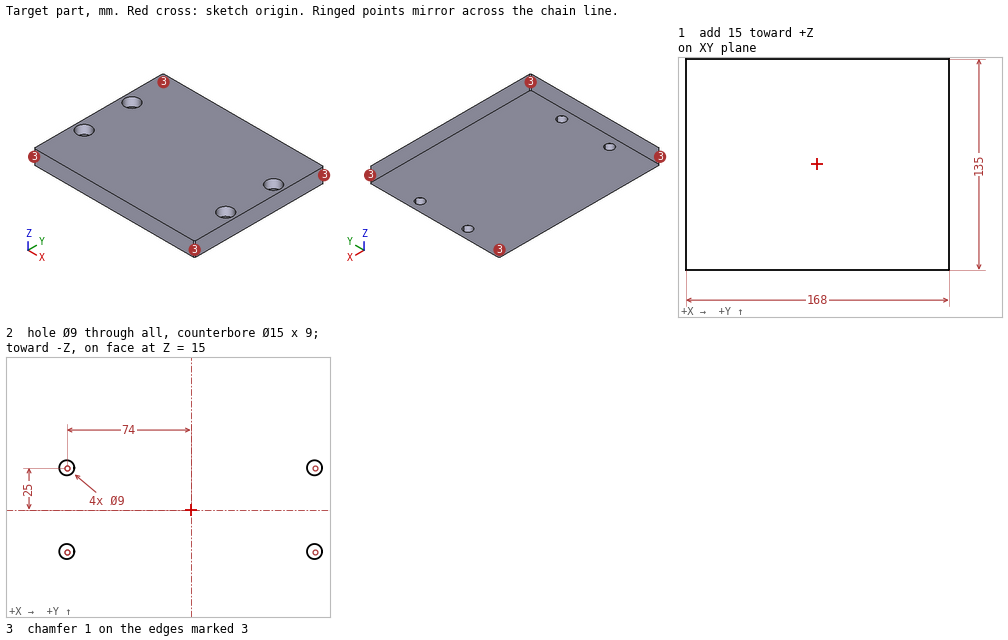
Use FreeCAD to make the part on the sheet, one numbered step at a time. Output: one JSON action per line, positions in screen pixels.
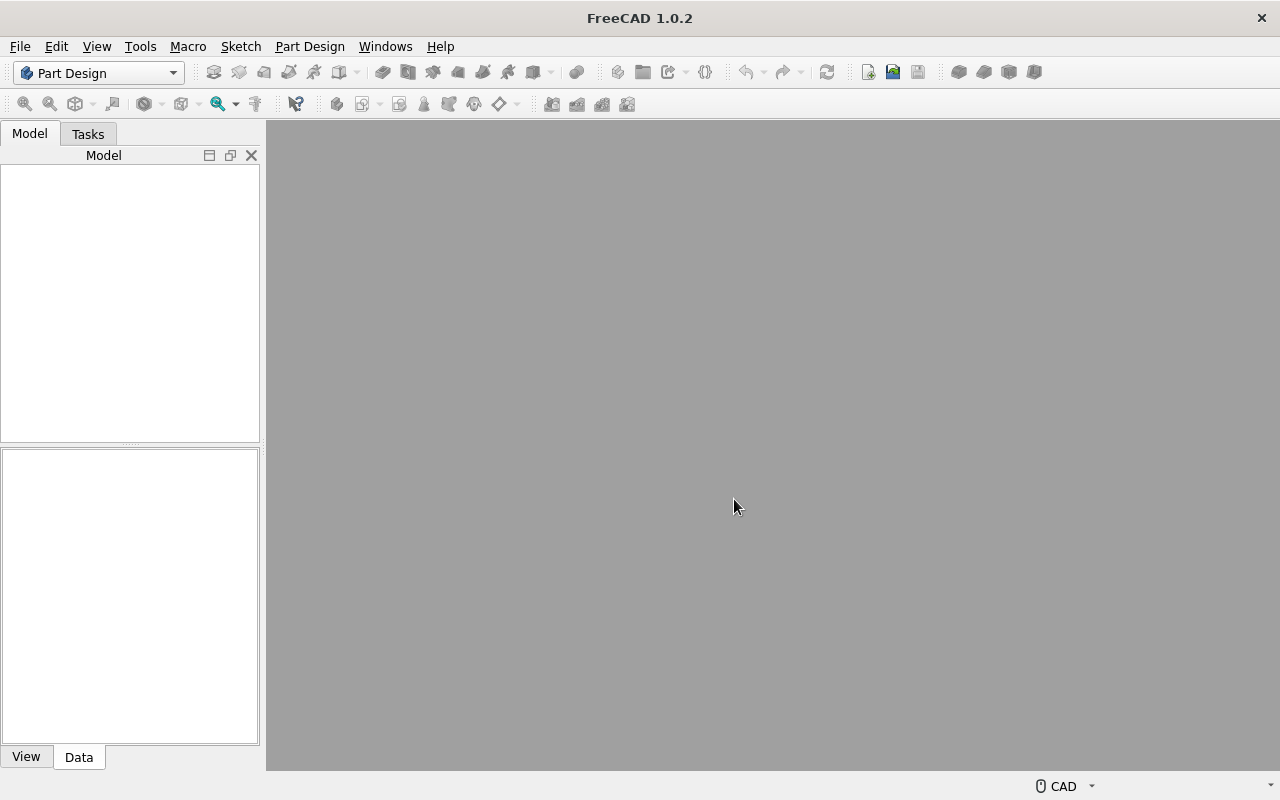
{"action": "key", "text": "ctrl+n"}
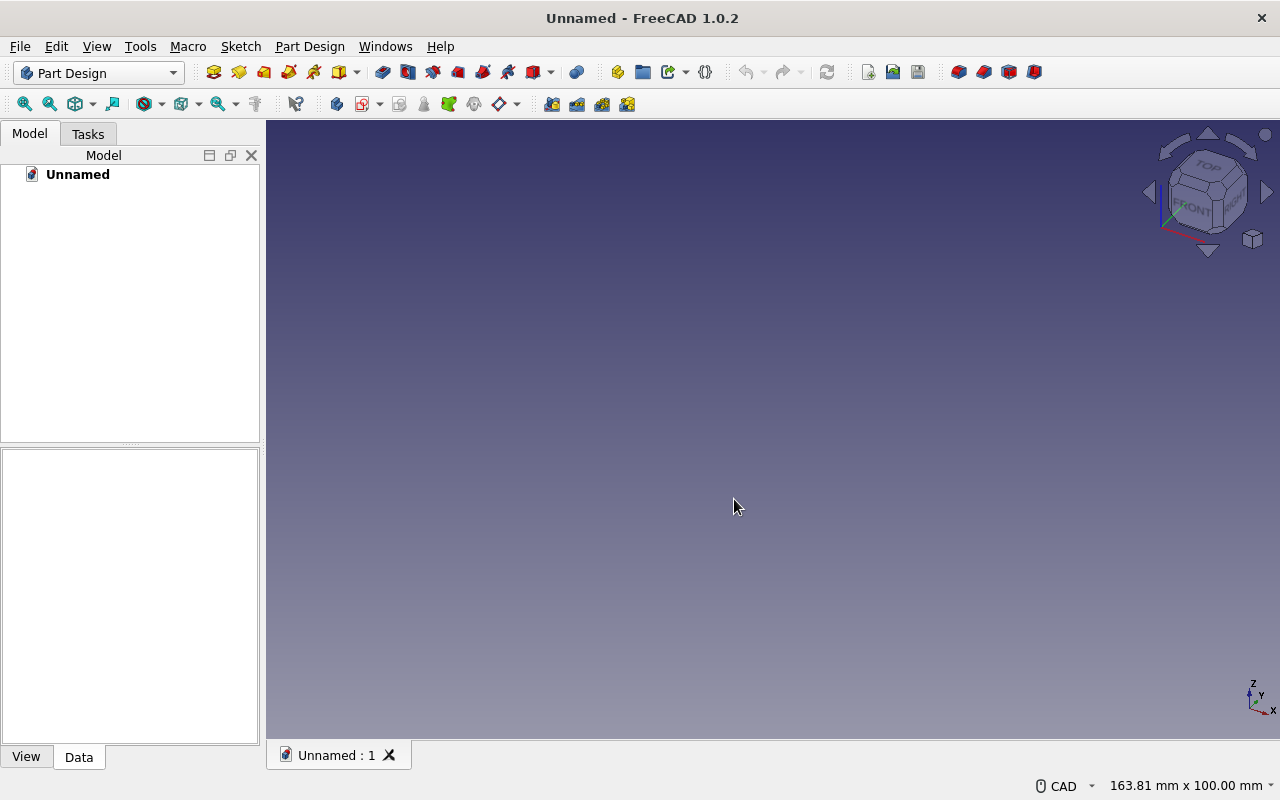
{"action": "left_click", "coordinate": [362, 104]}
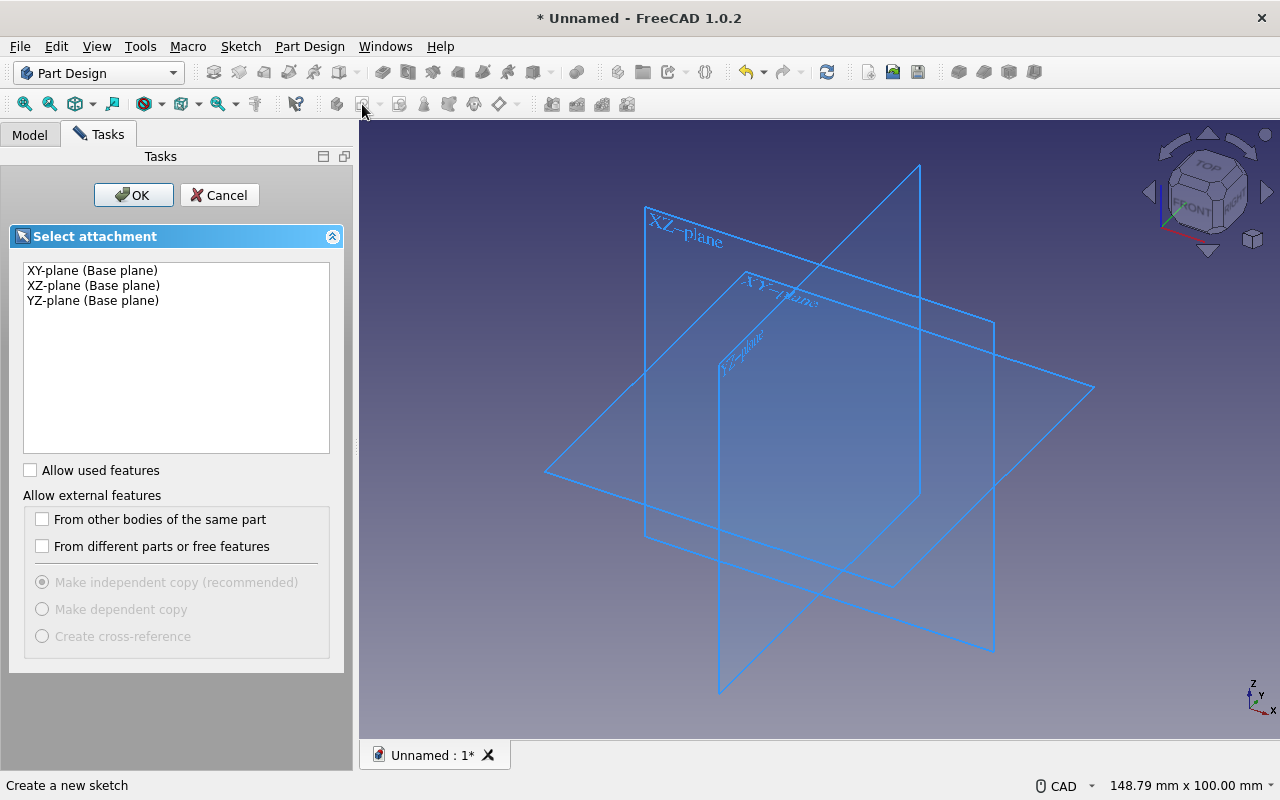
{"action": "left_click", "coordinate": [84, 270]}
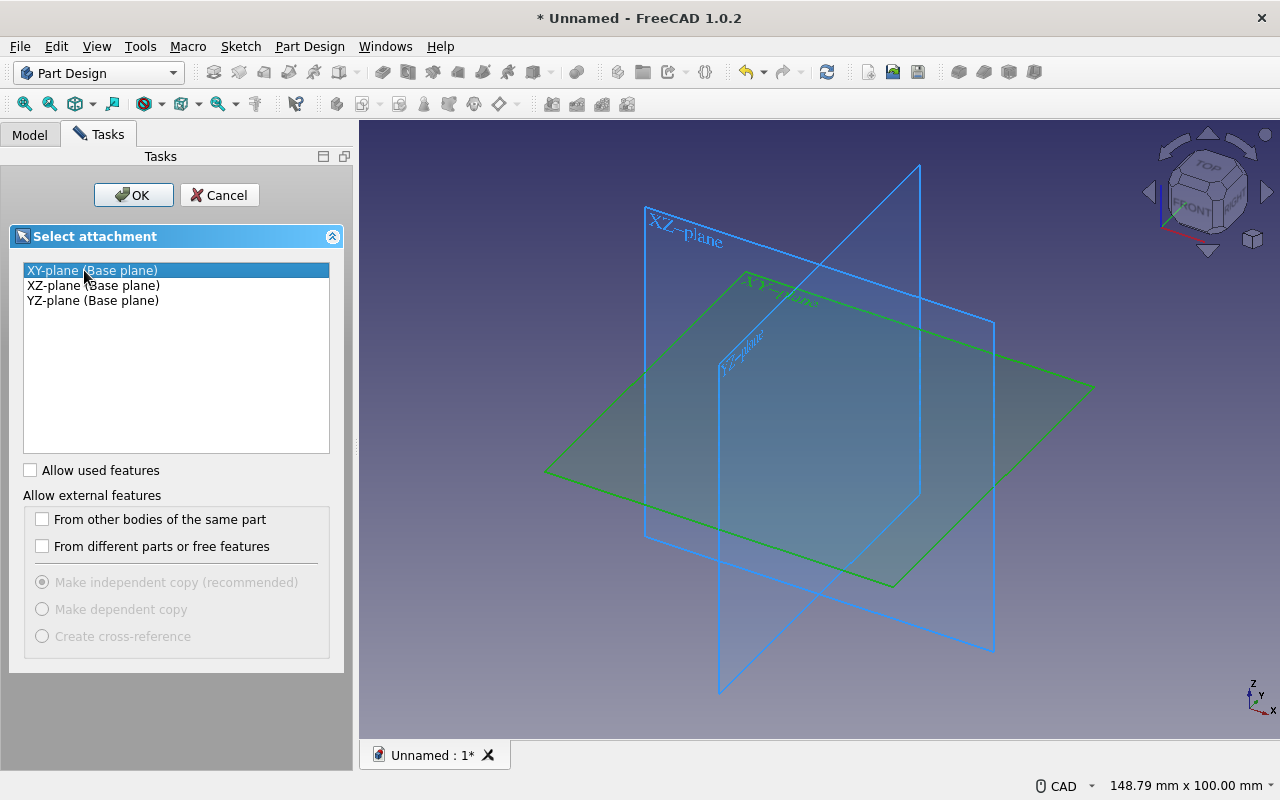
{"action": "left_click", "coordinate": [134, 195]}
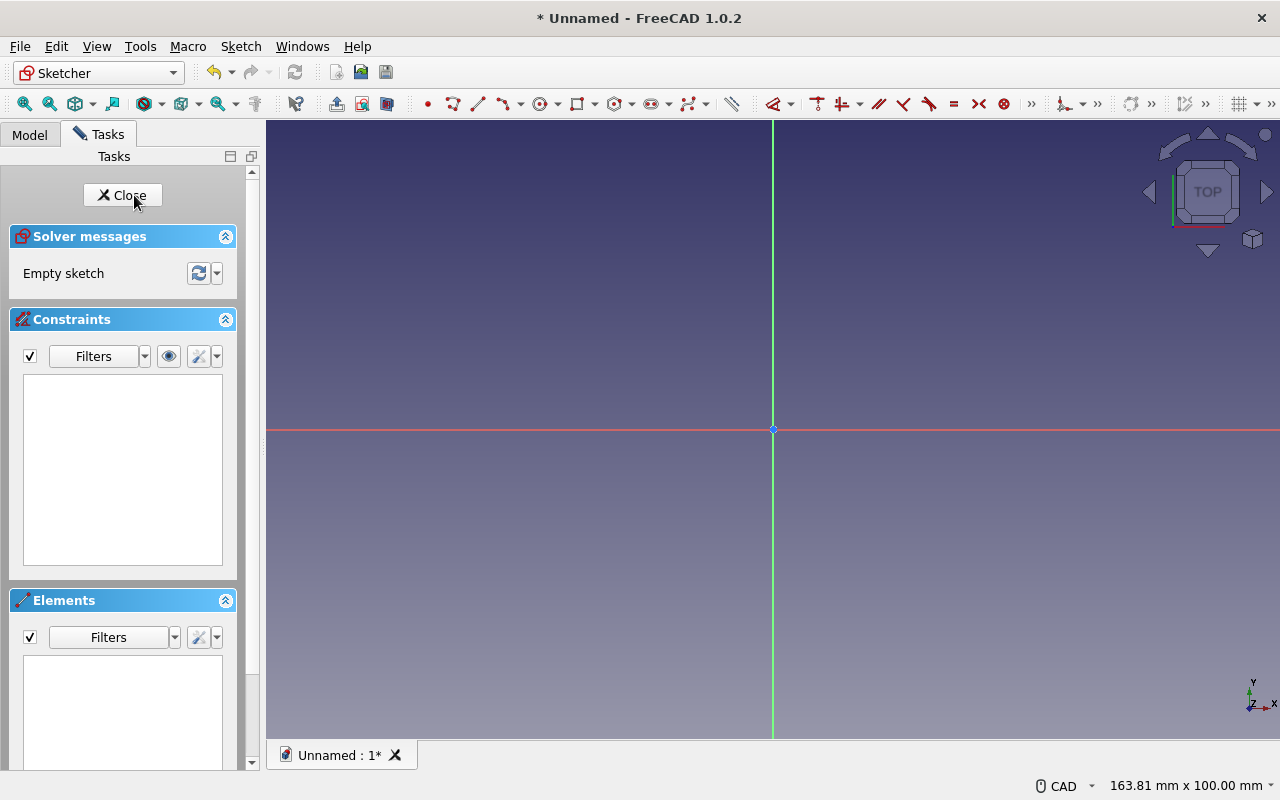
{"action": "scroll", "coordinate": [649, 430], "scroll_direction": "down", "scroll_amount": 4}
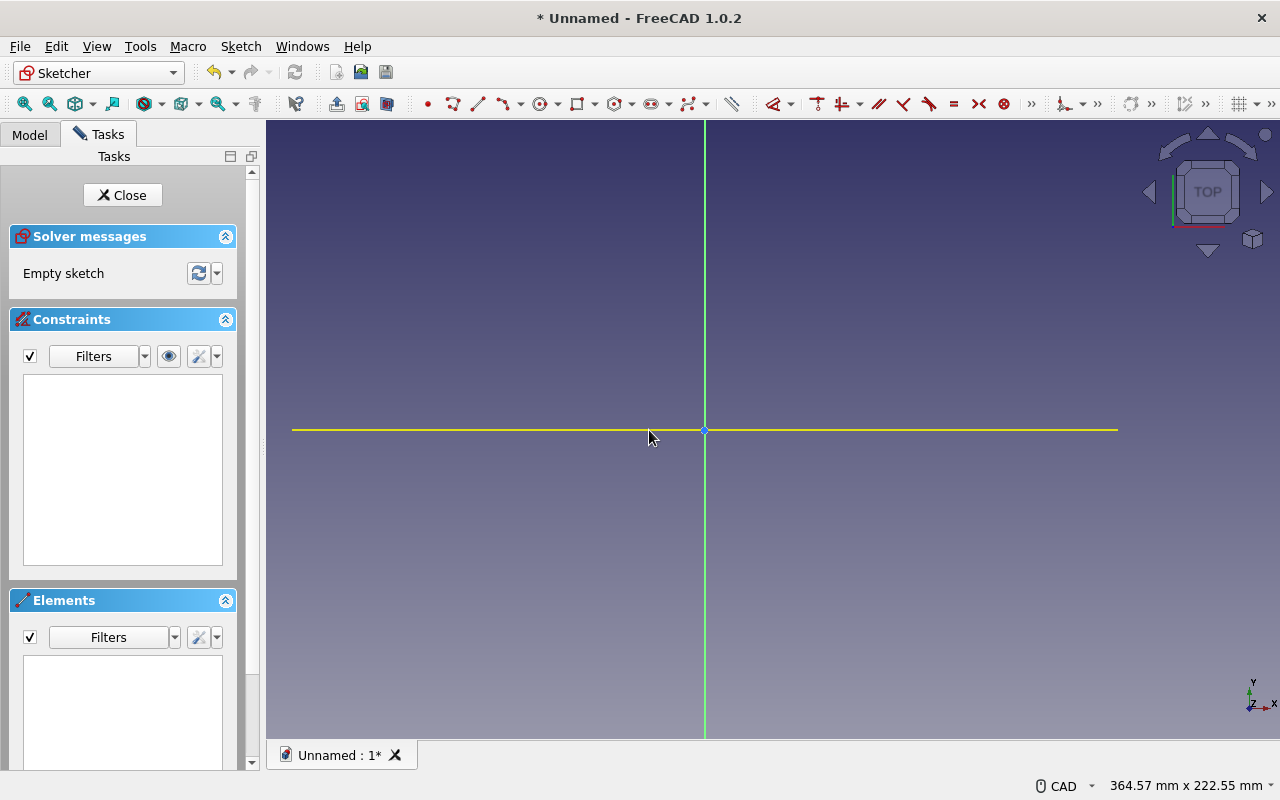
{"action": "key", "text": "g v"}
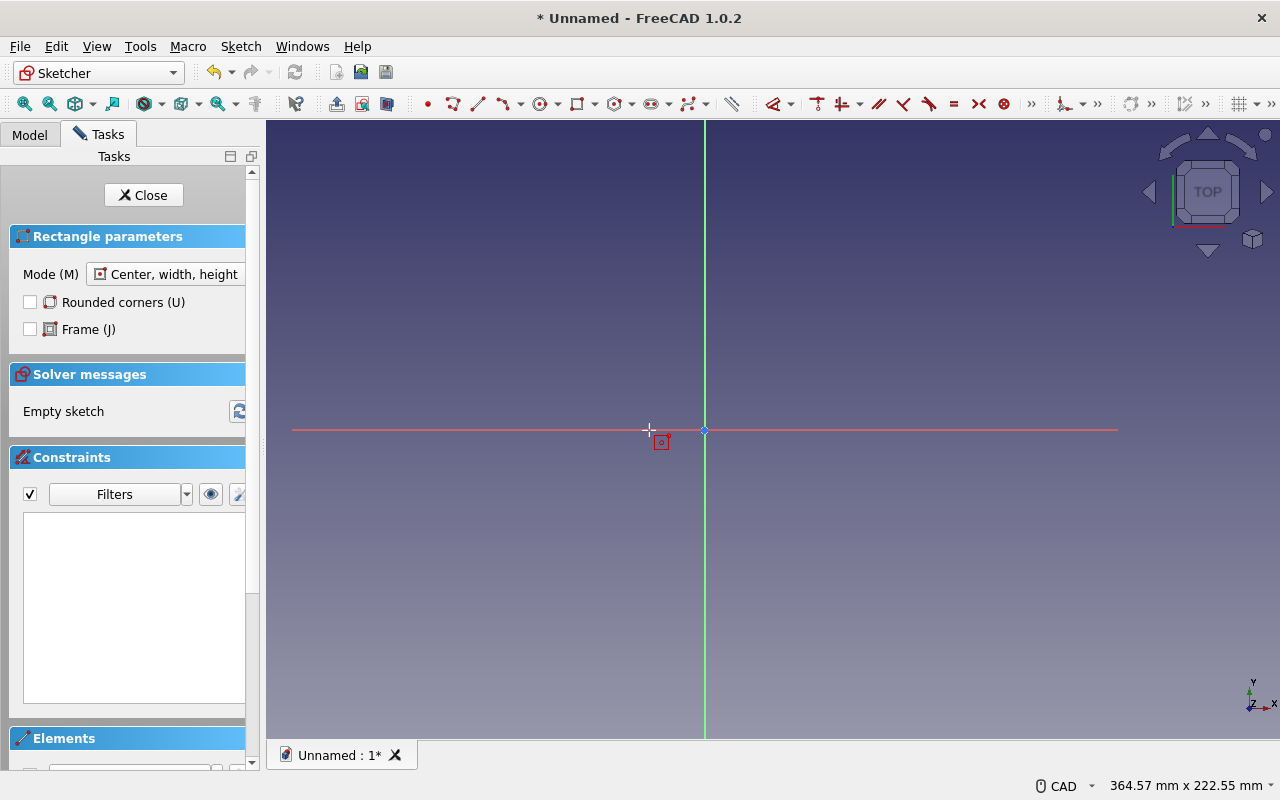
{"action": "left_click", "coordinate": [705, 430]}
{"action": "left_click", "coordinate": [939, 242]}
{"action": "key", "text": "Escape"}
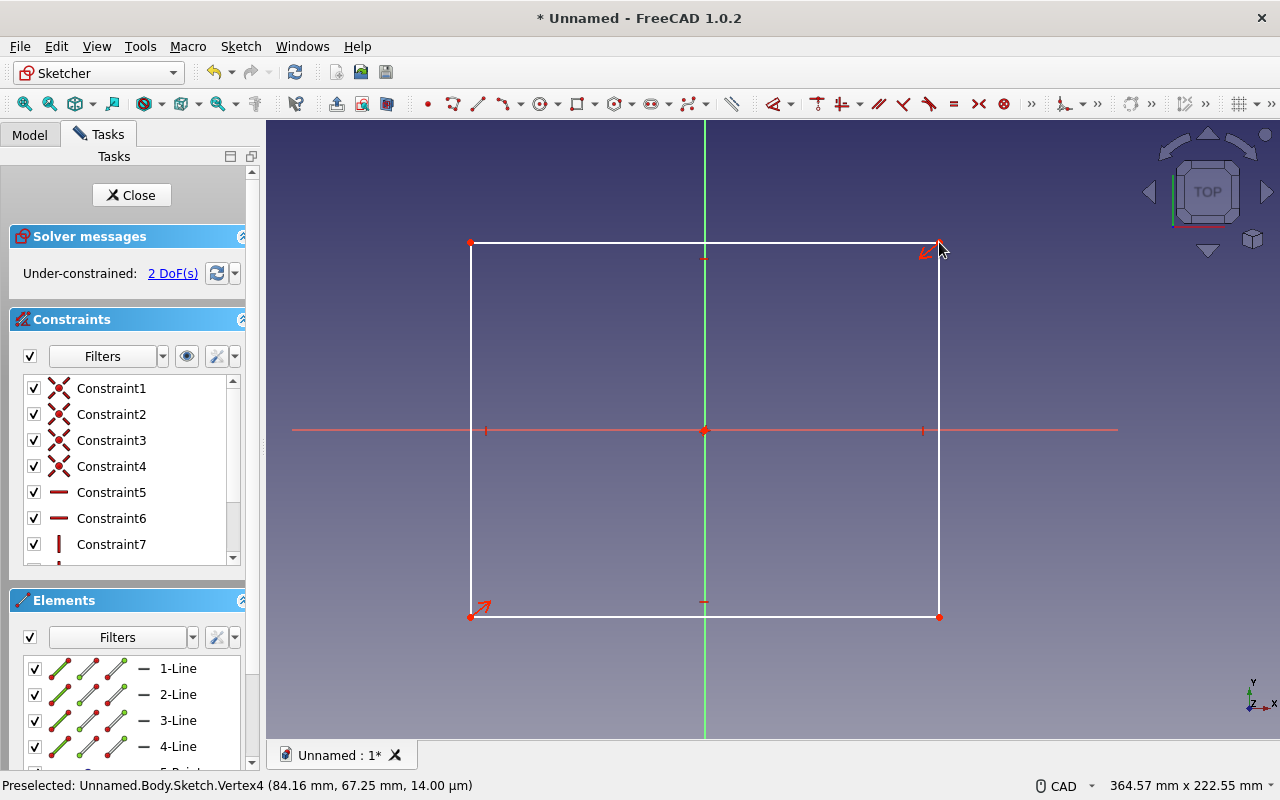
{"action": "key", "text": "d"}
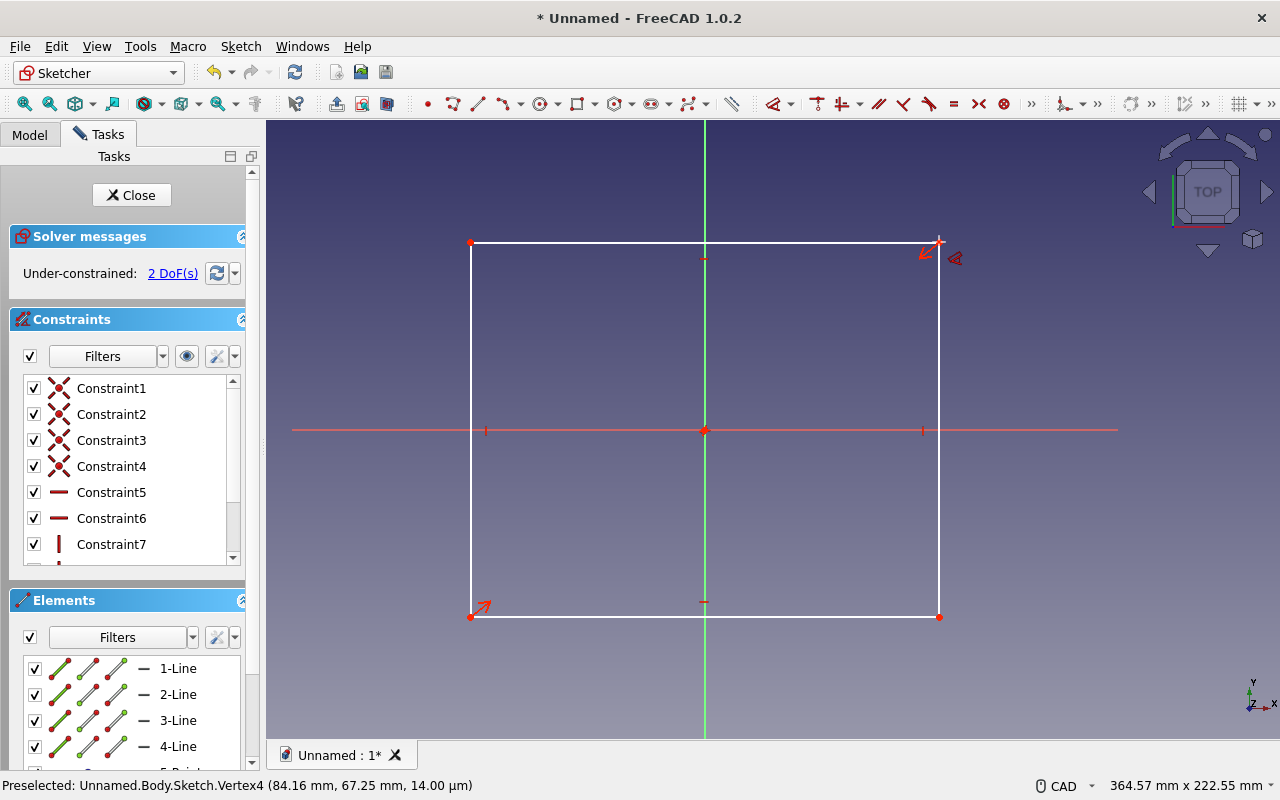
{"action": "left_click", "coordinate": [611, 617]}
{"action": "left_click", "coordinate": [597, 651]}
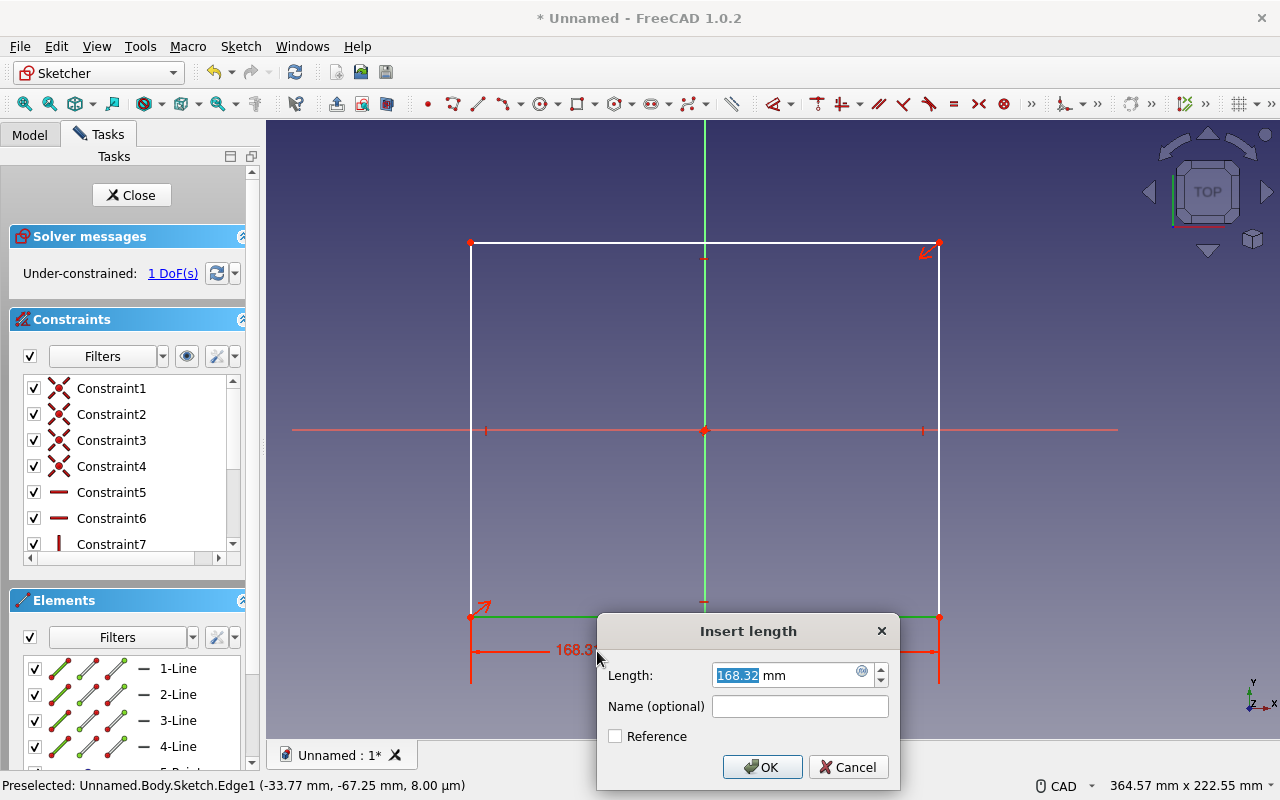
{"action": "type", "text": "168"}
{"action": "key", "text": "Return"}